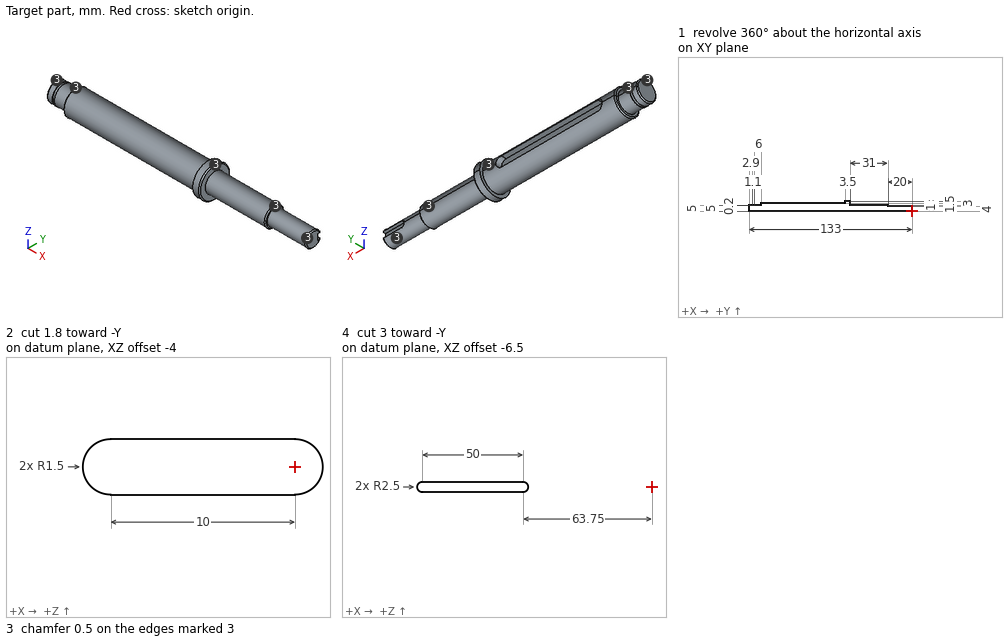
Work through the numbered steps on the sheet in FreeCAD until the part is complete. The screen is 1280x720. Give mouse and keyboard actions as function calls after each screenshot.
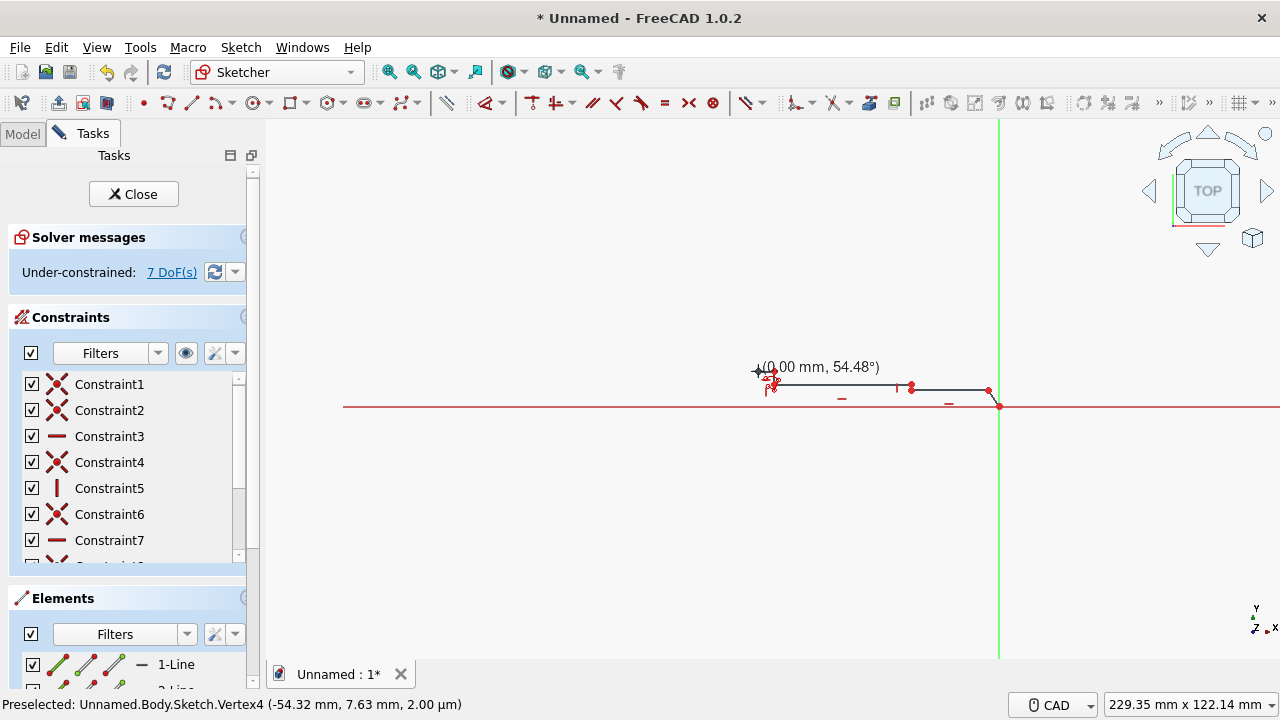
scroll(758, 378, up, 5)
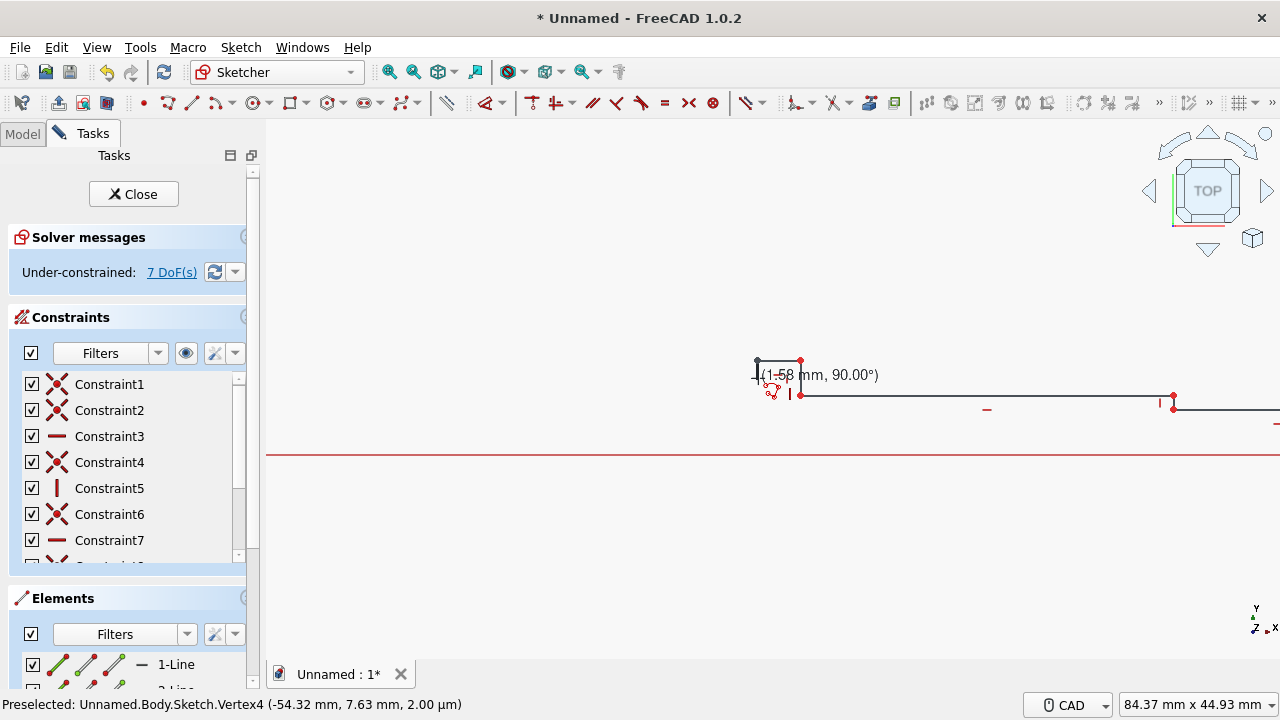
click(757, 377)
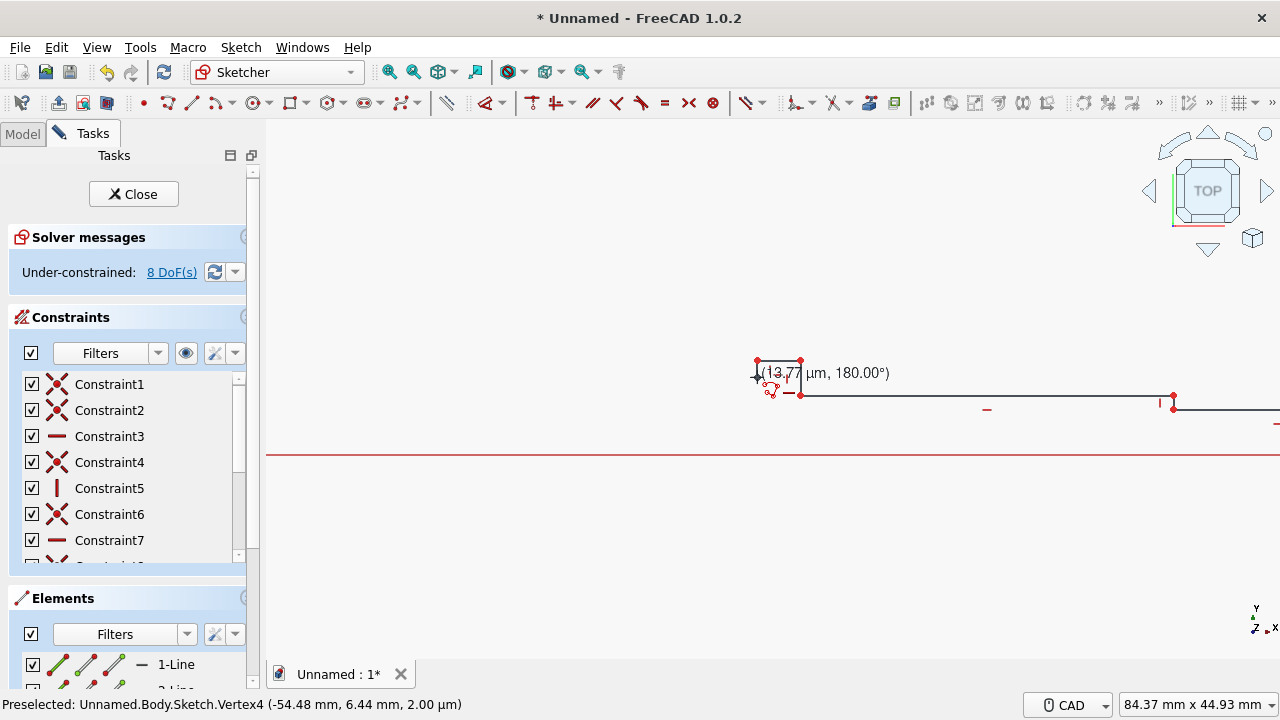
scroll(757, 378, down, 5)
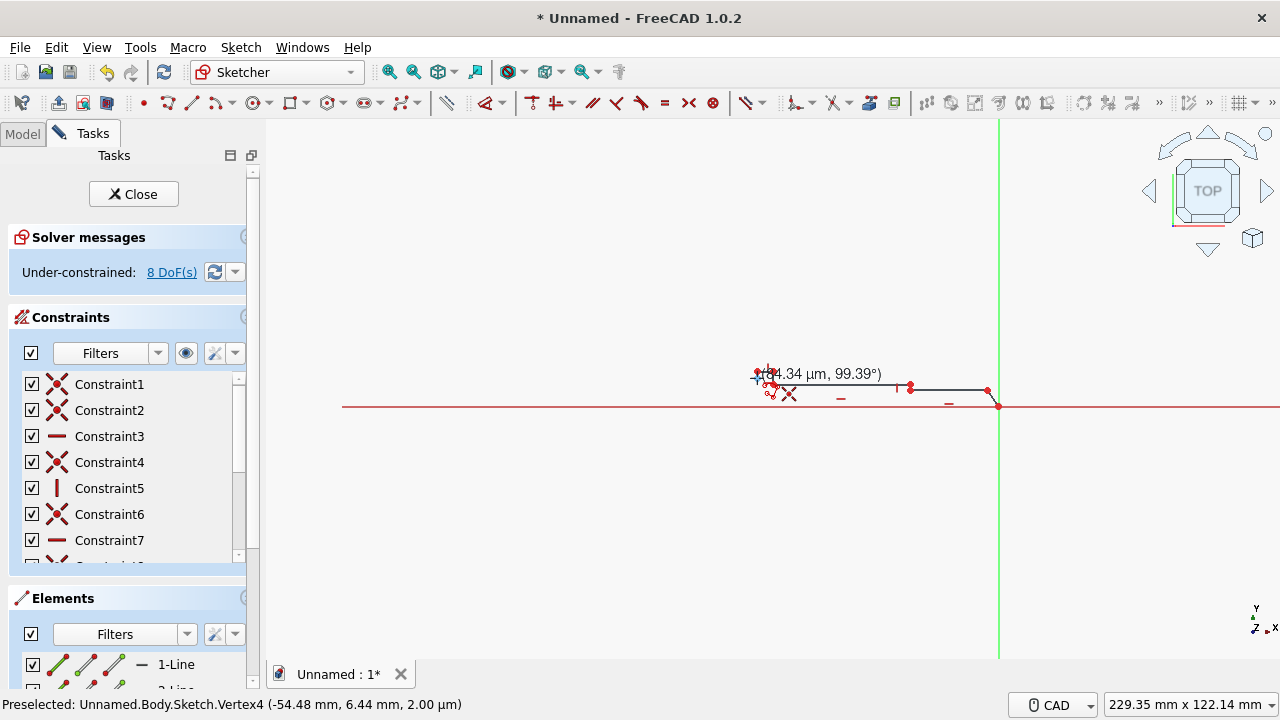
click(455, 378)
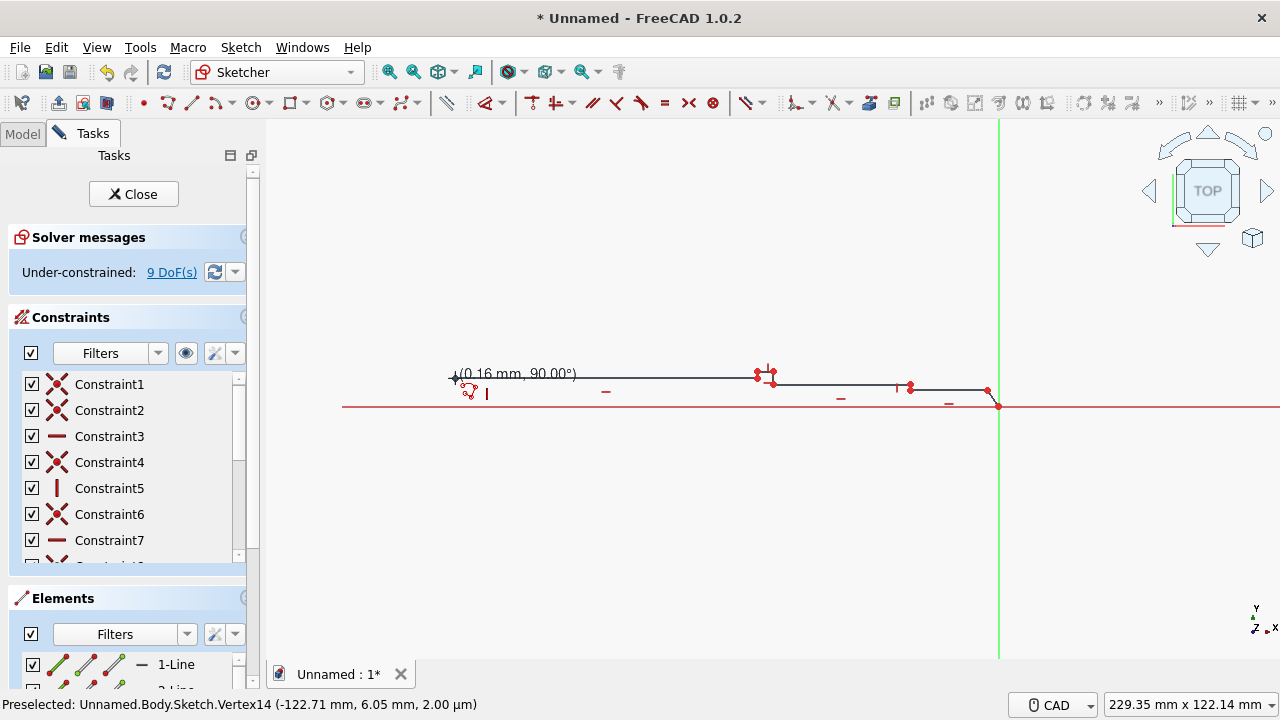
scroll(455, 385, up, 5)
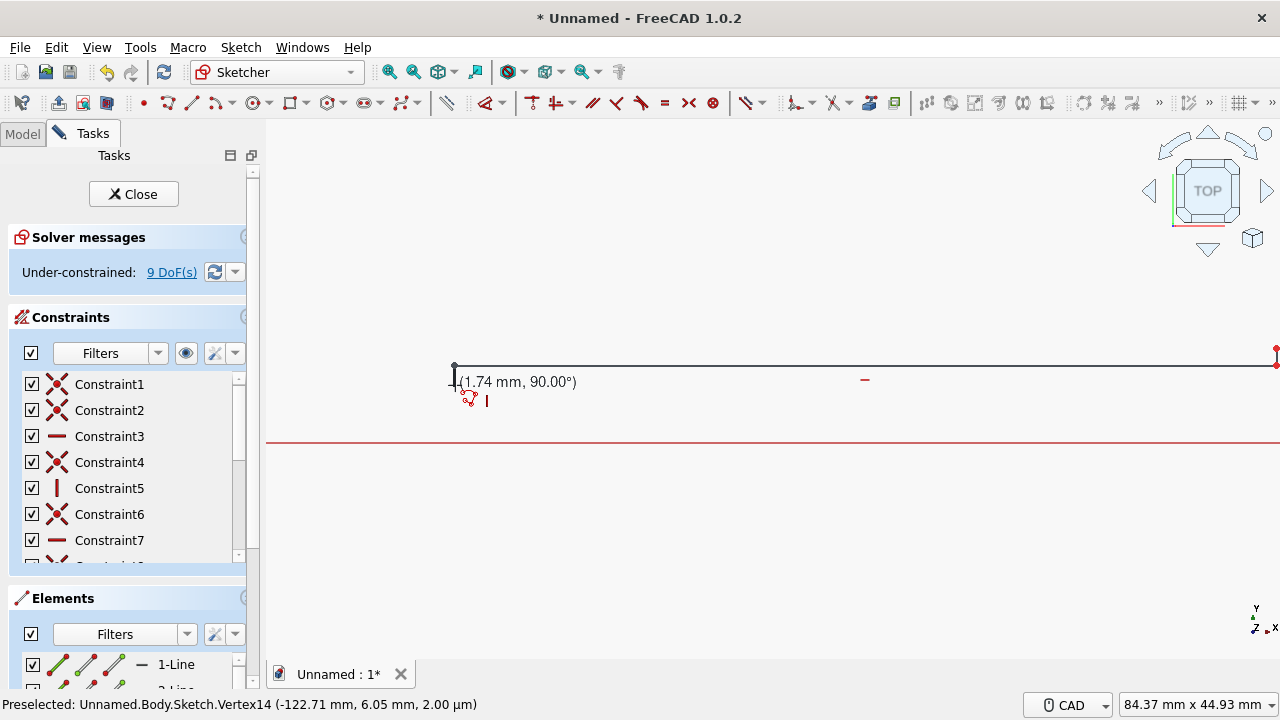
click(455, 383)
click(382, 383)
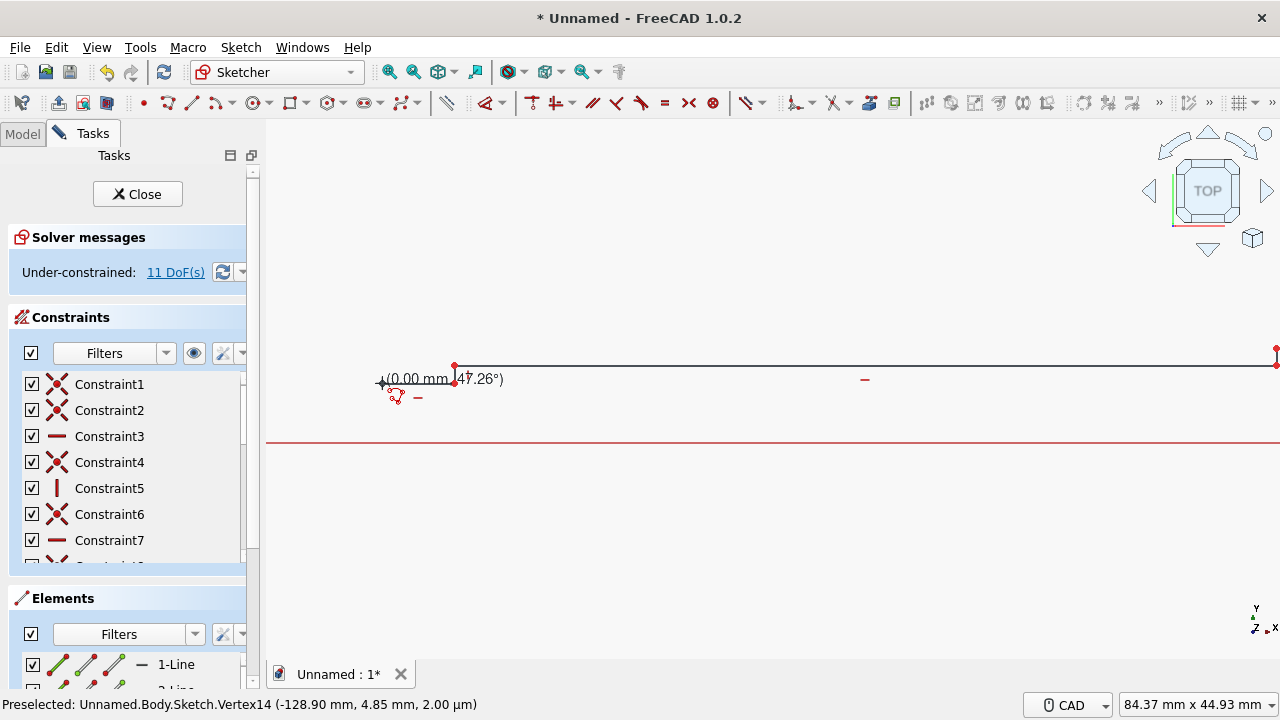
scroll(382, 386, up, 10)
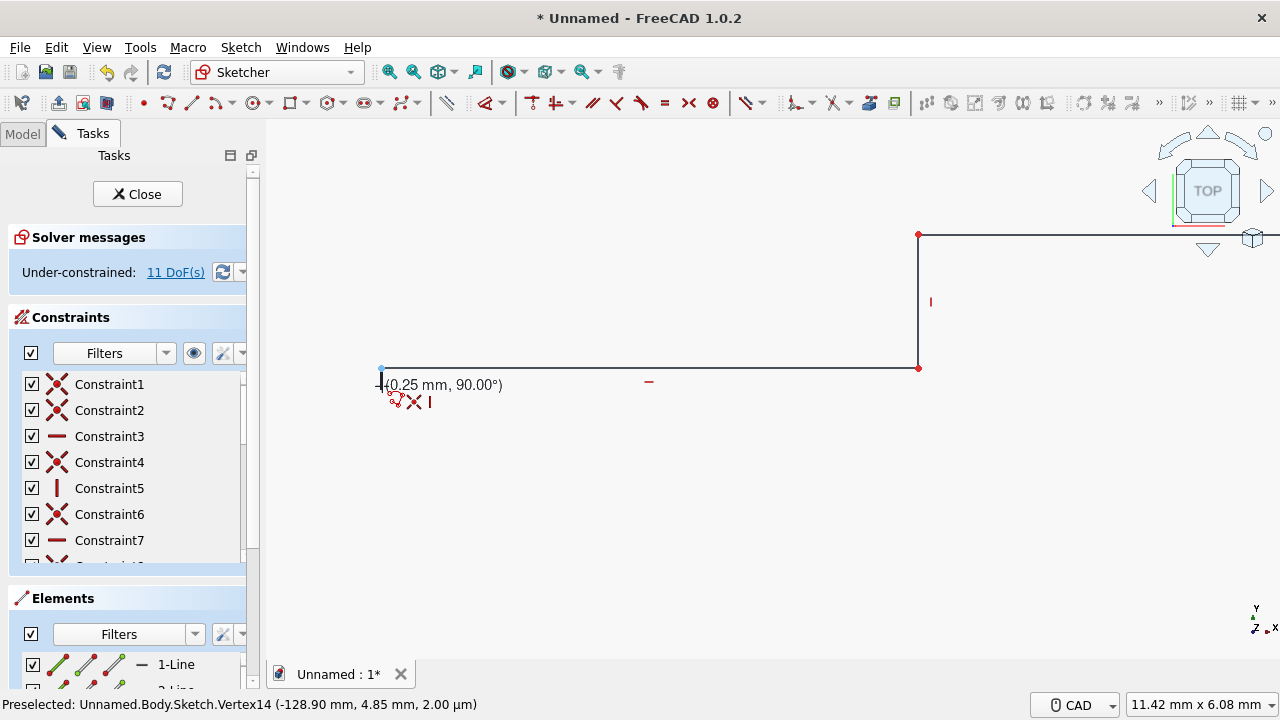
click(381, 380)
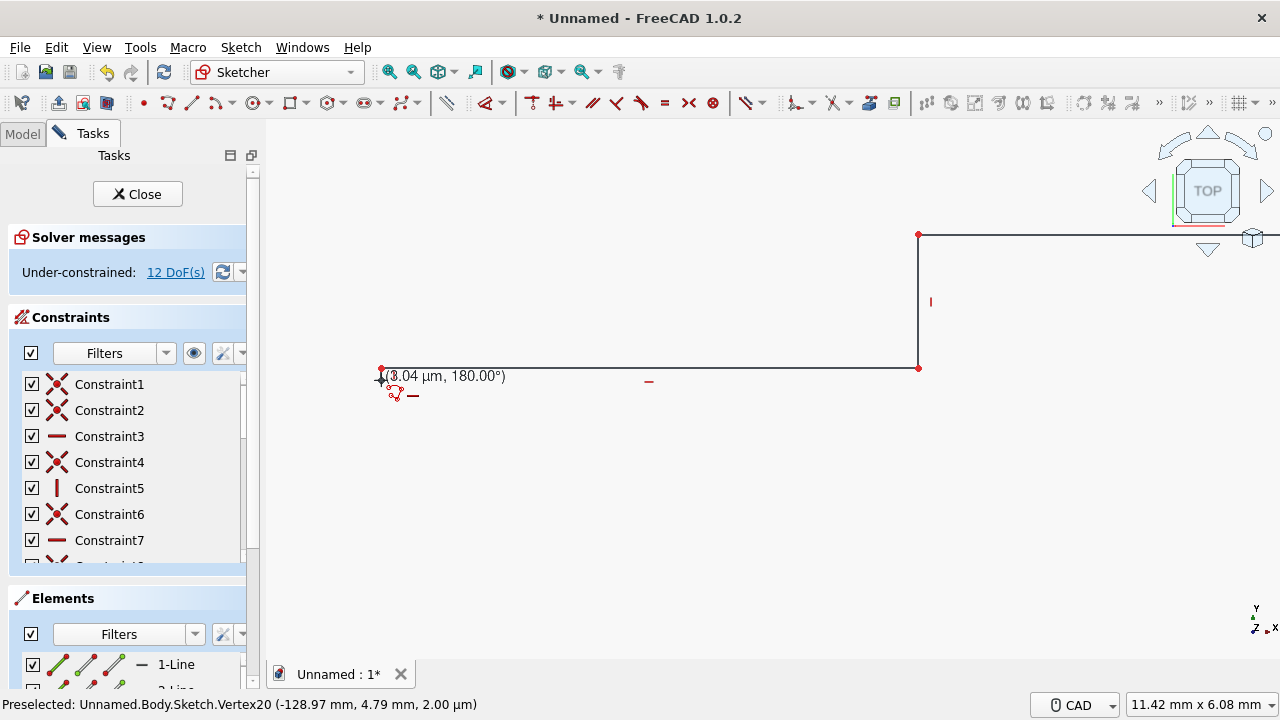
scroll(431, 386, down, 15)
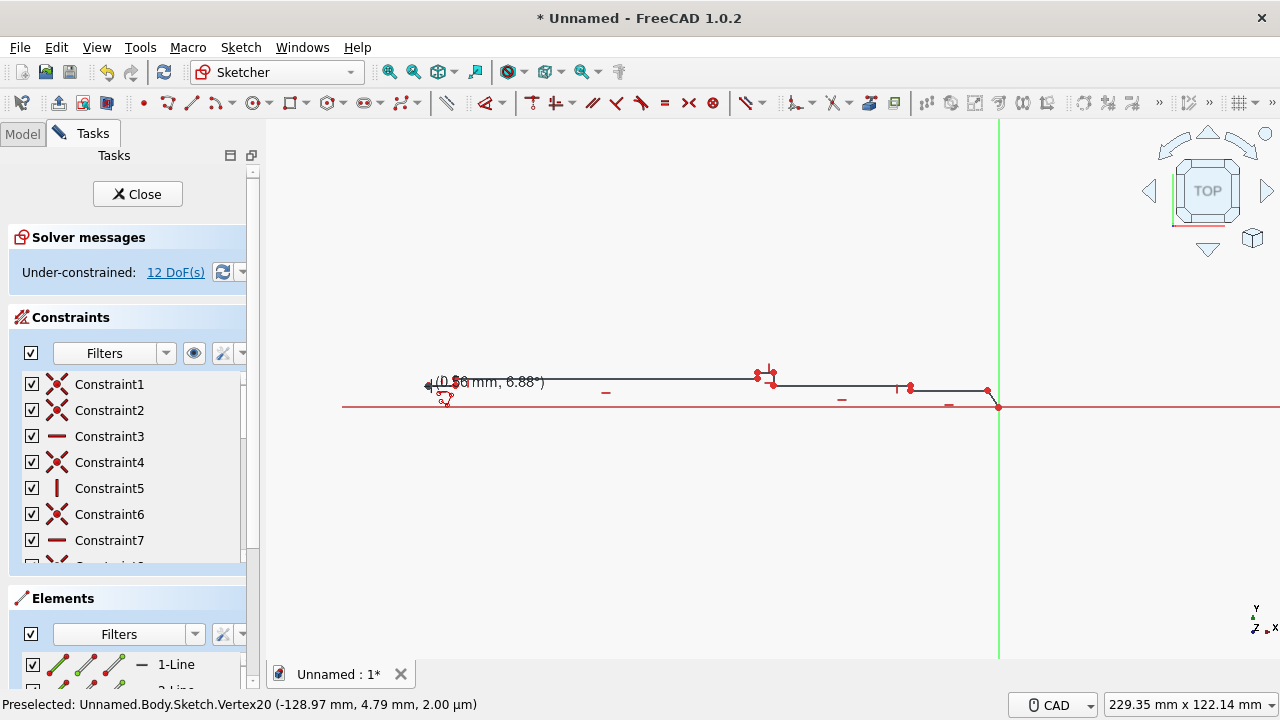
scroll(424, 386, up, 6)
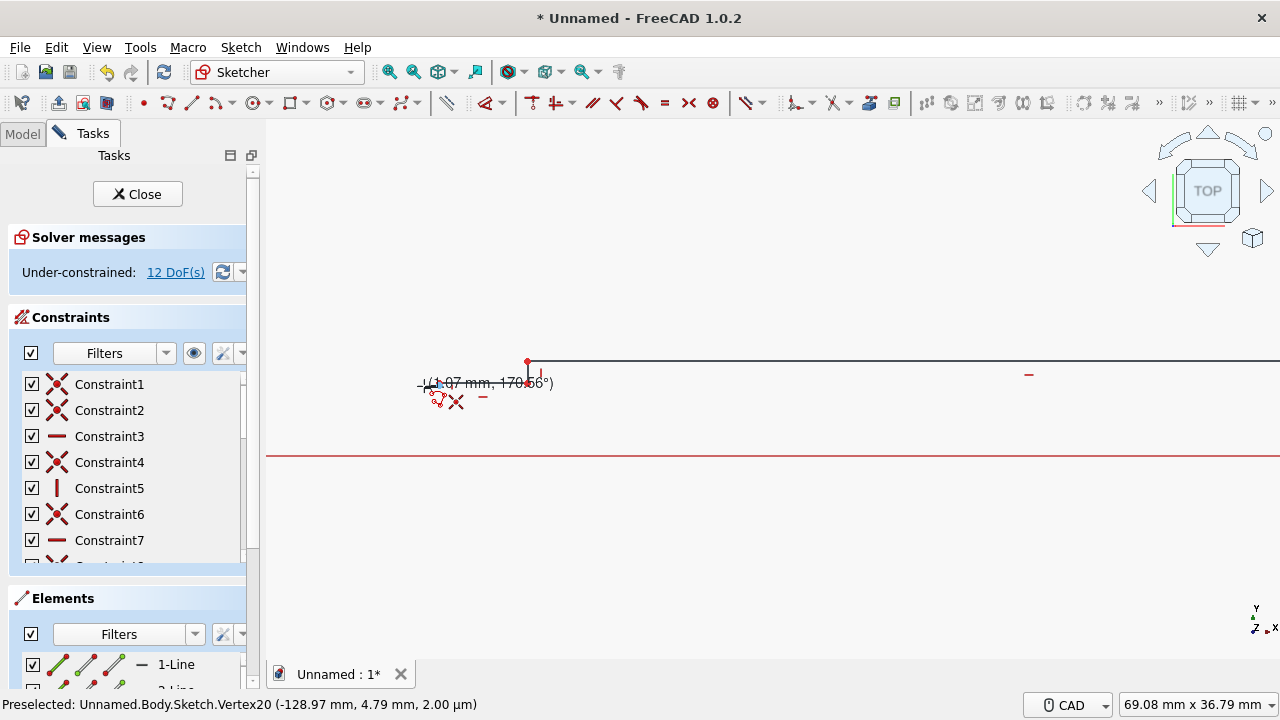
click(423, 385)